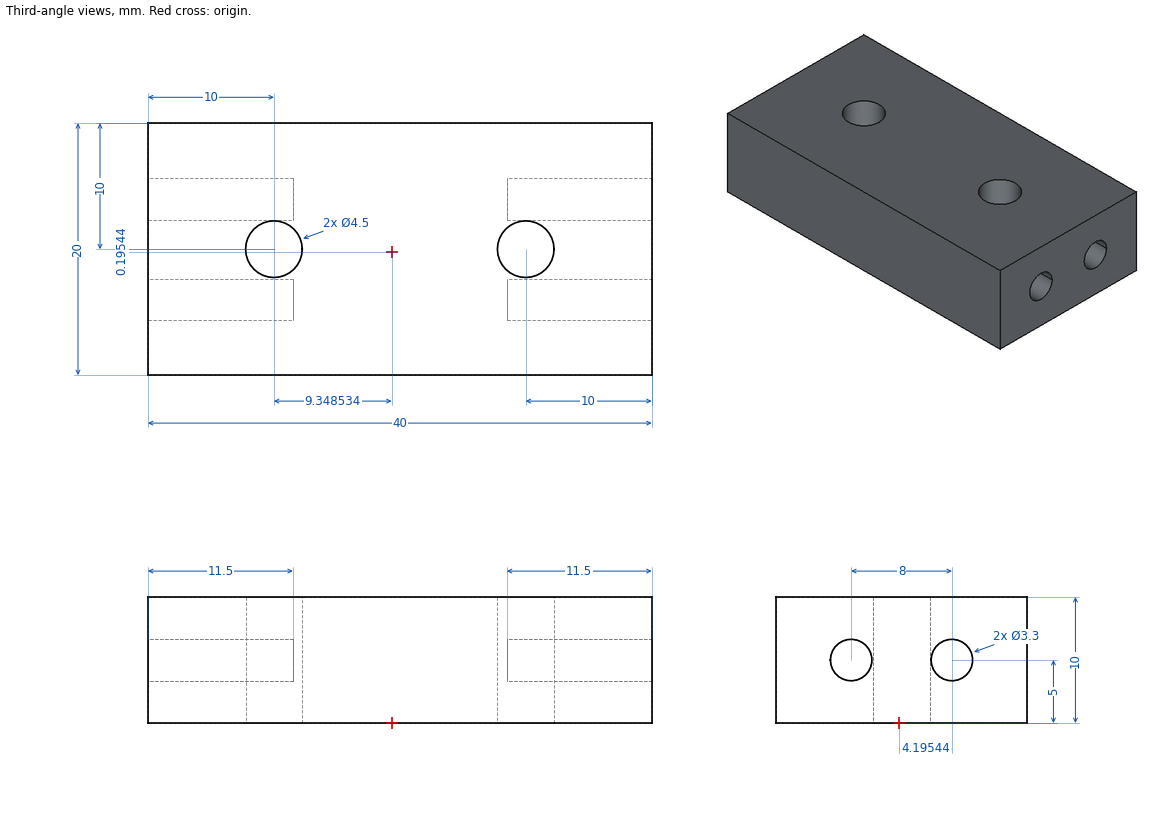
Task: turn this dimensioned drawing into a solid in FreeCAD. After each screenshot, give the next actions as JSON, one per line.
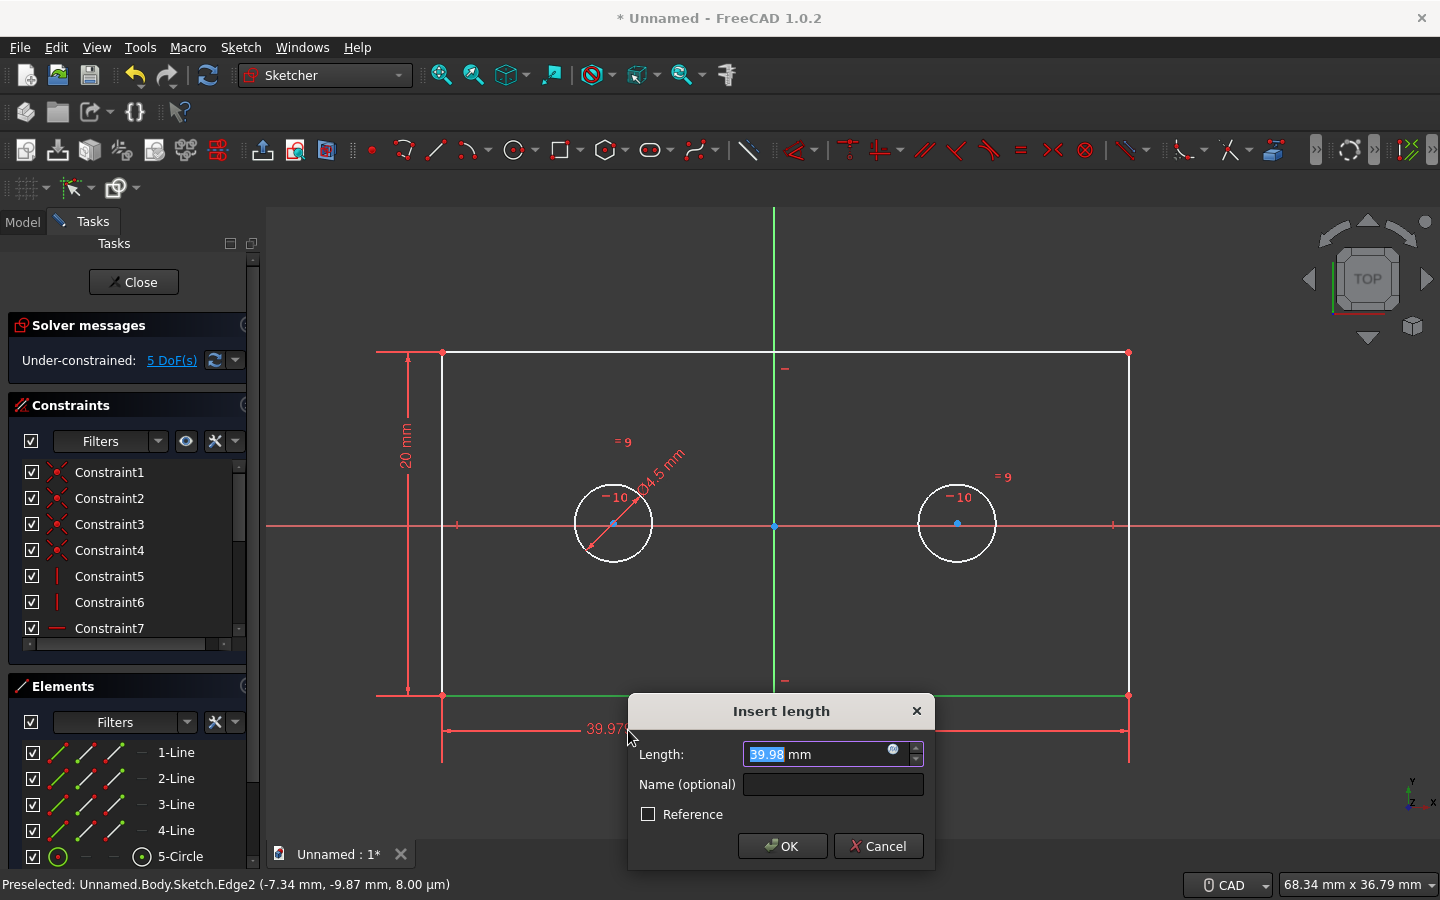
{"action": "type", "text": "40"}
{"action": "key", "text": "Return"}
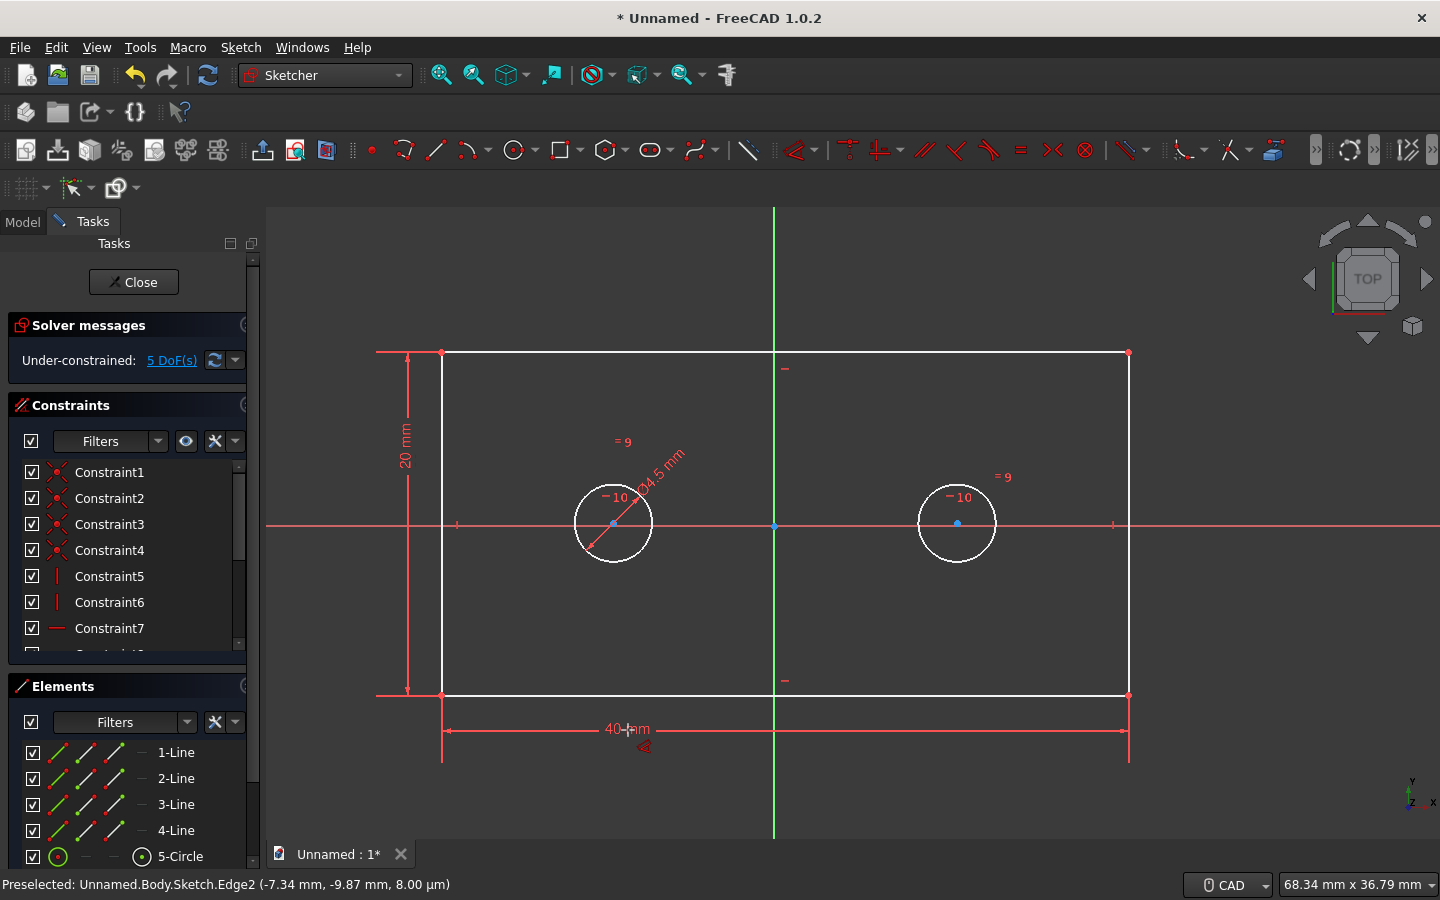
{"action": "left_click", "coordinate": [442, 352]}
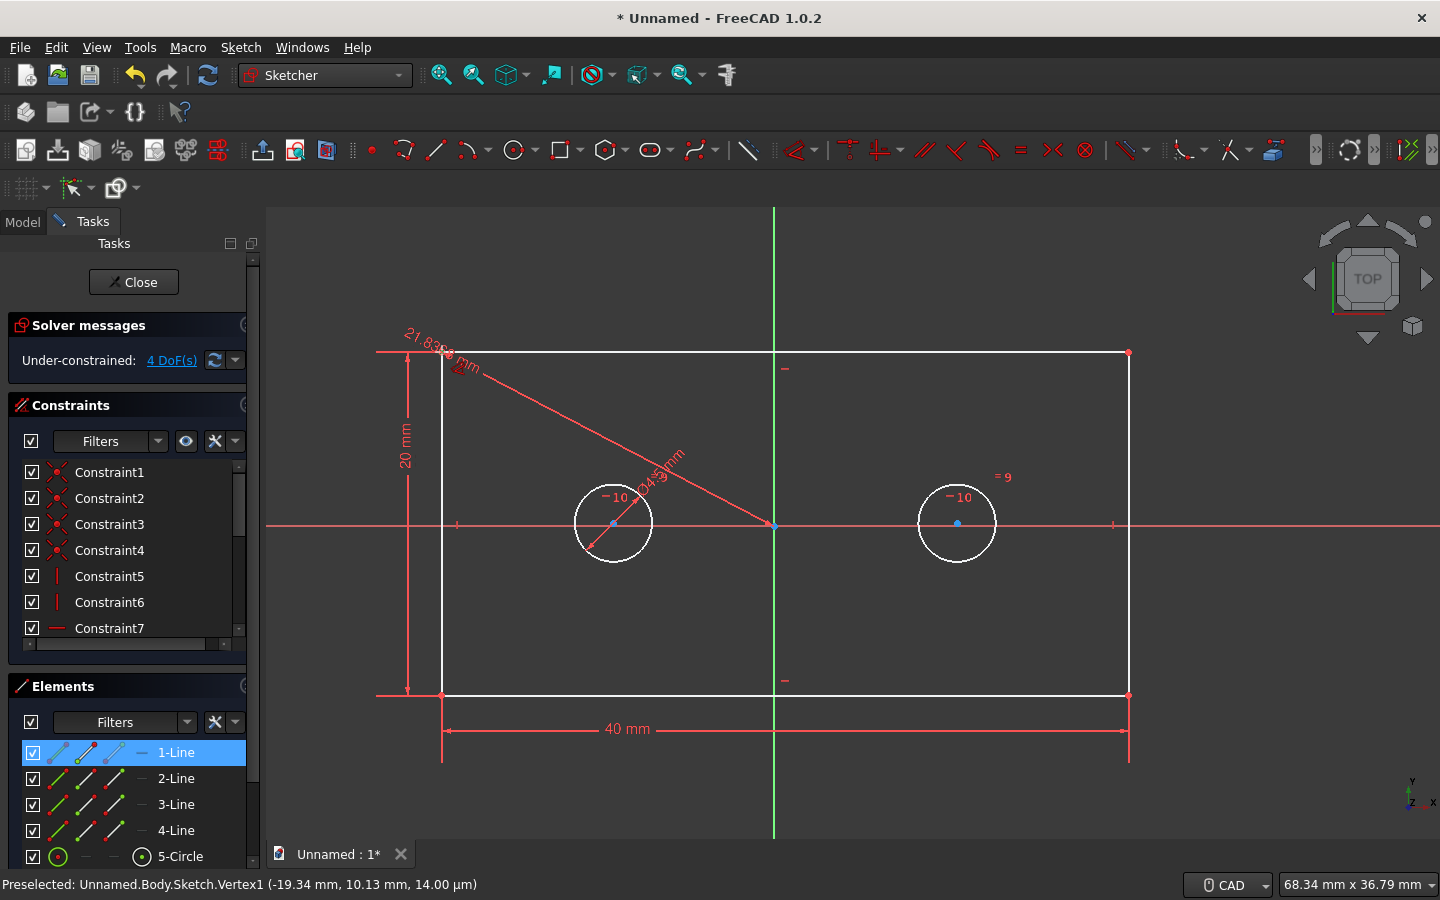
{"action": "left_click", "coordinate": [613, 523]}
{"action": "left_click", "coordinate": [528, 318]}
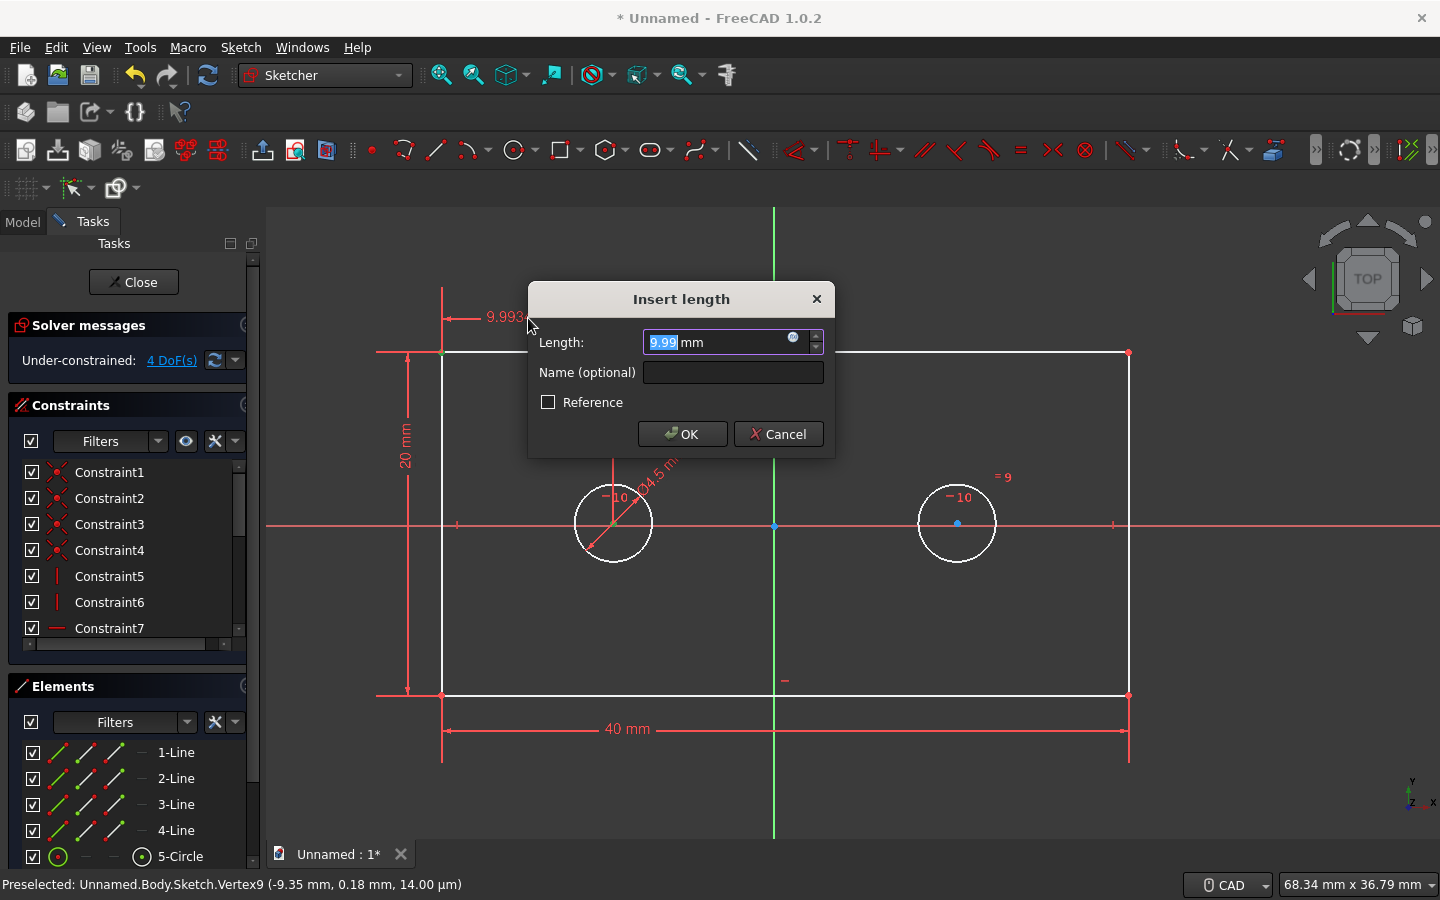
{"action": "type", "text": "10"}
{"action": "key", "text": "Return"}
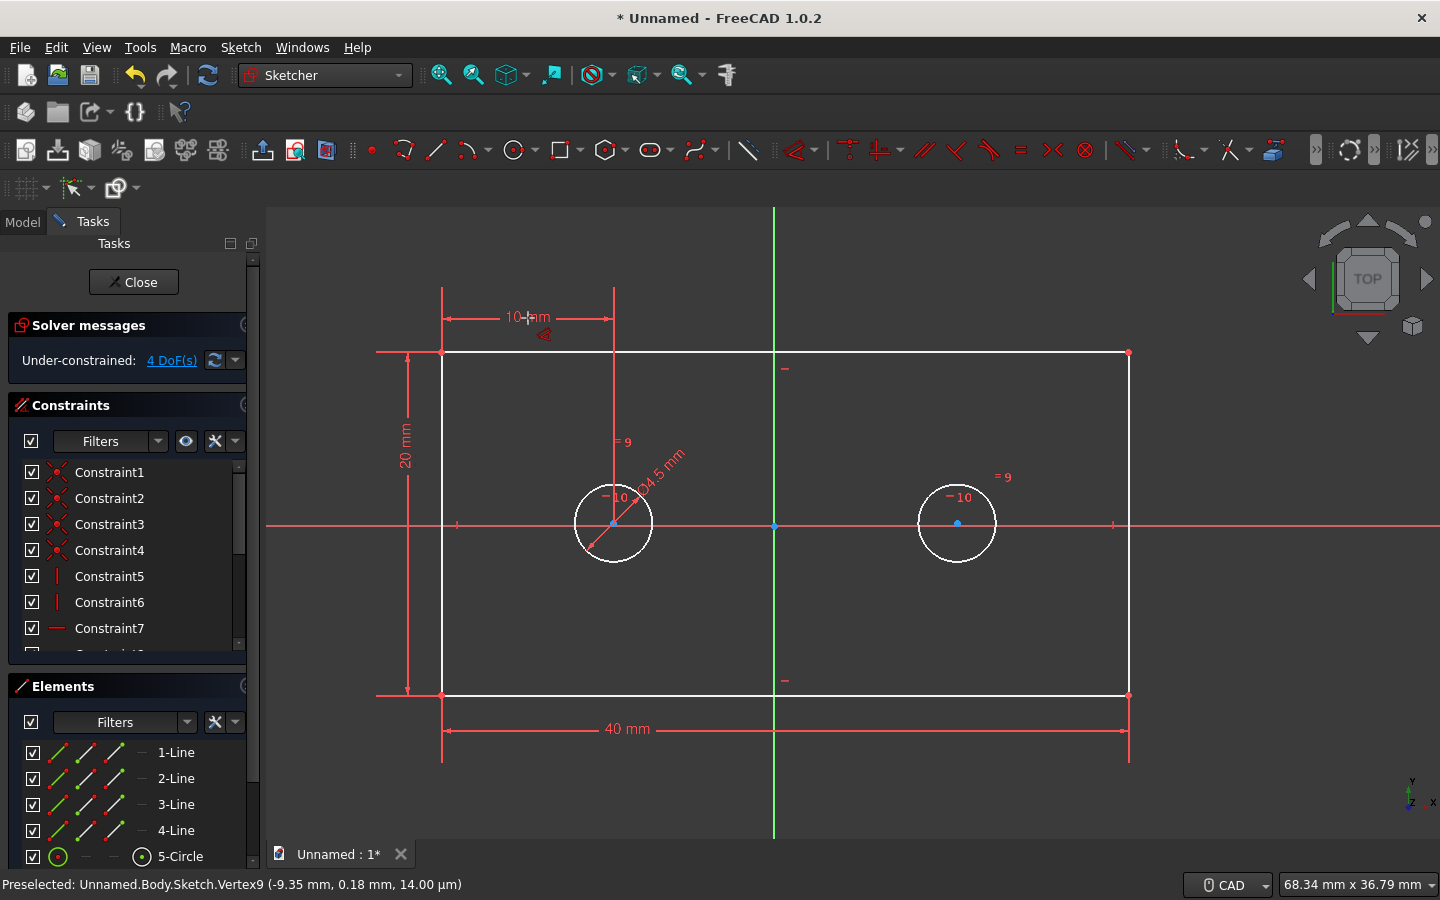
{"action": "left_click", "coordinate": [442, 352]}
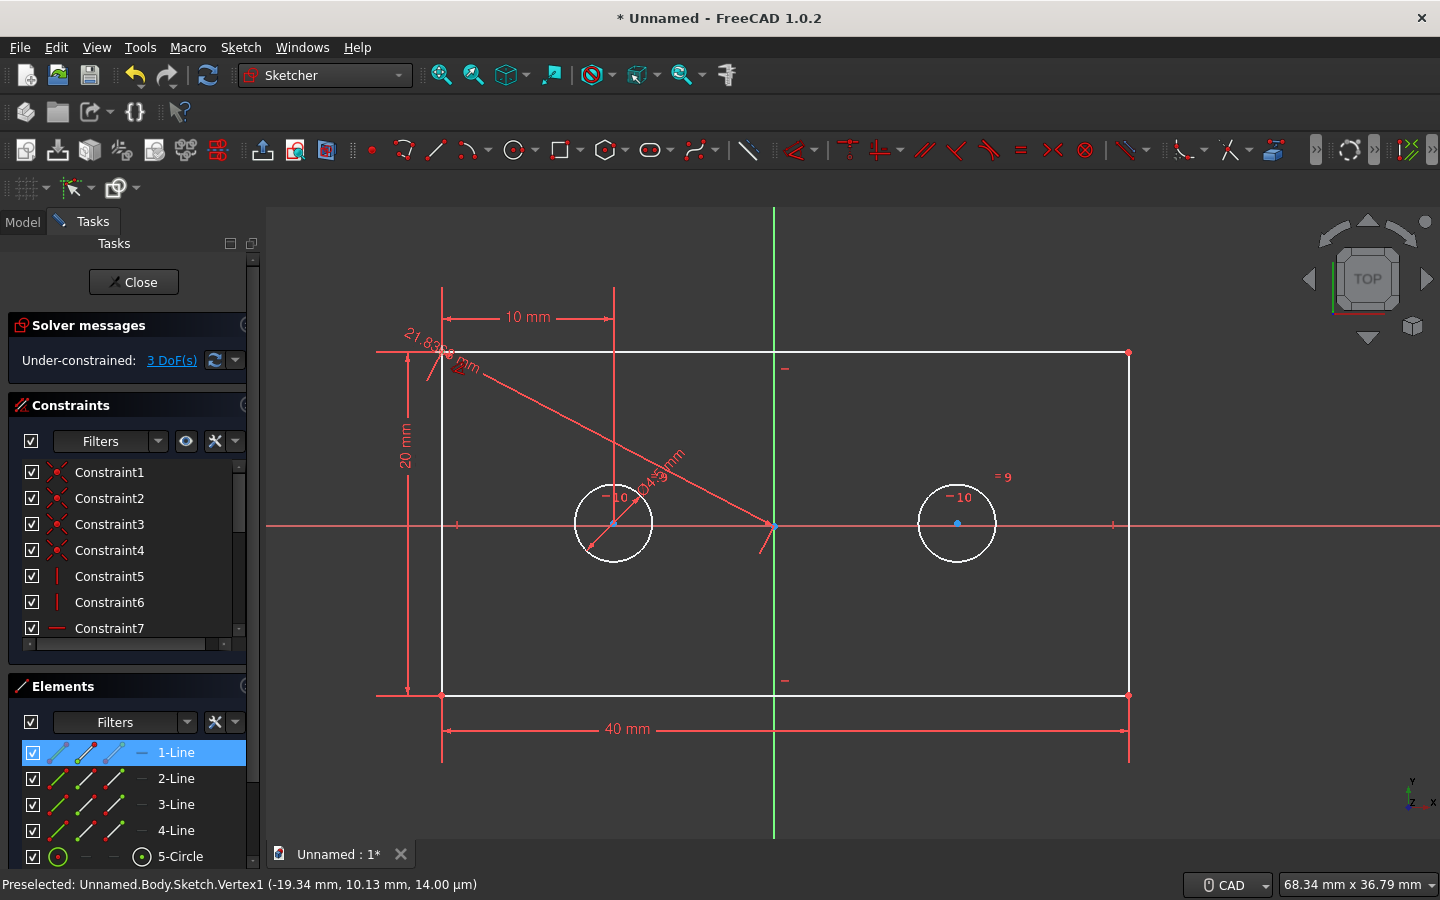
{"action": "left_click", "coordinate": [614, 523]}
{"action": "left_click", "coordinate": [408, 398]}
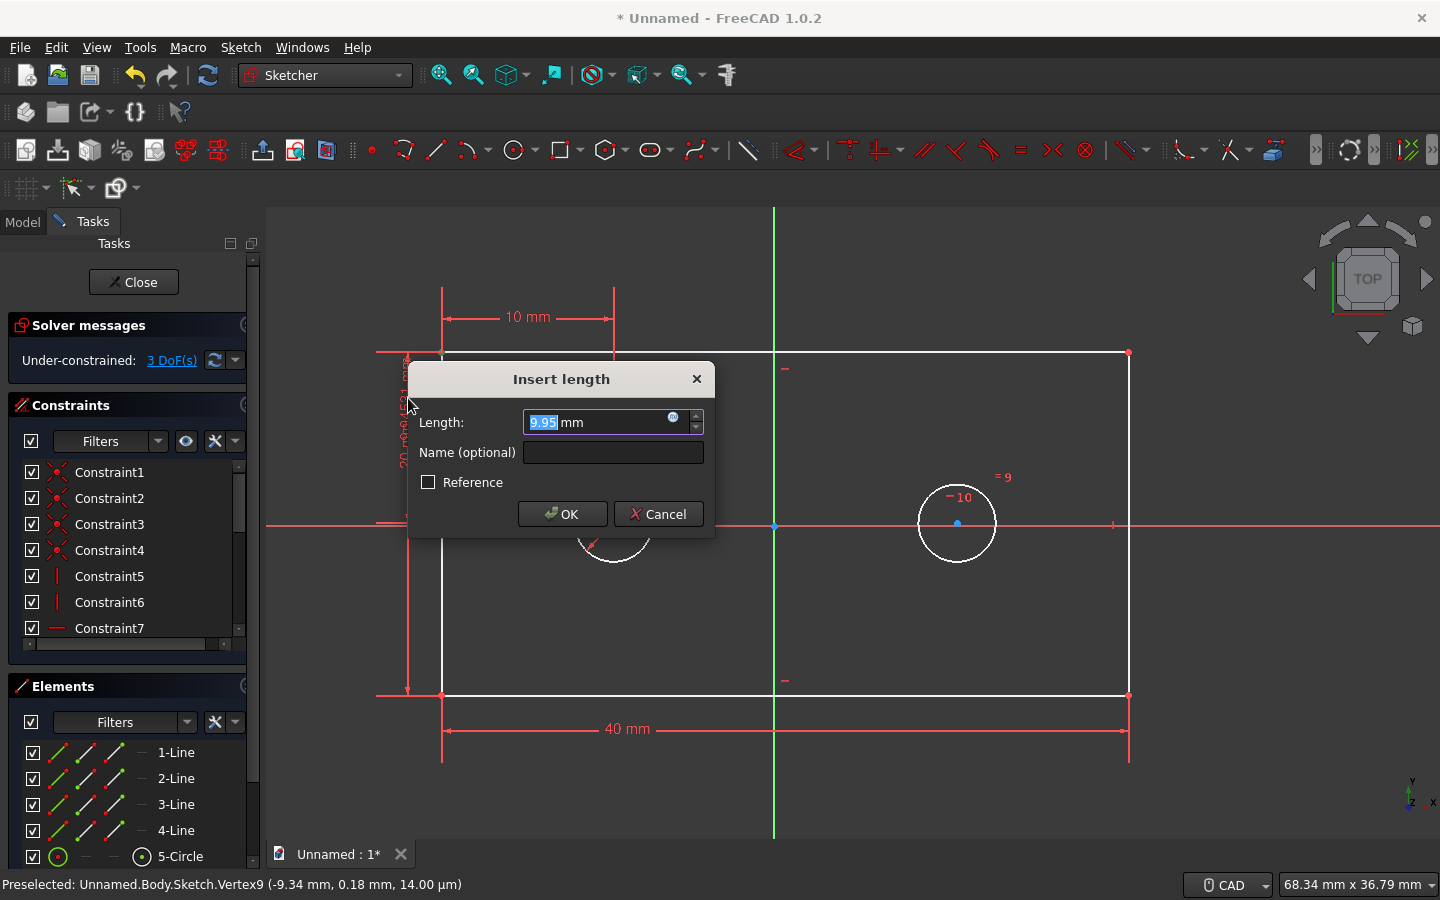
{"action": "type", "text": "10"}
{"action": "key", "text": "Return"}